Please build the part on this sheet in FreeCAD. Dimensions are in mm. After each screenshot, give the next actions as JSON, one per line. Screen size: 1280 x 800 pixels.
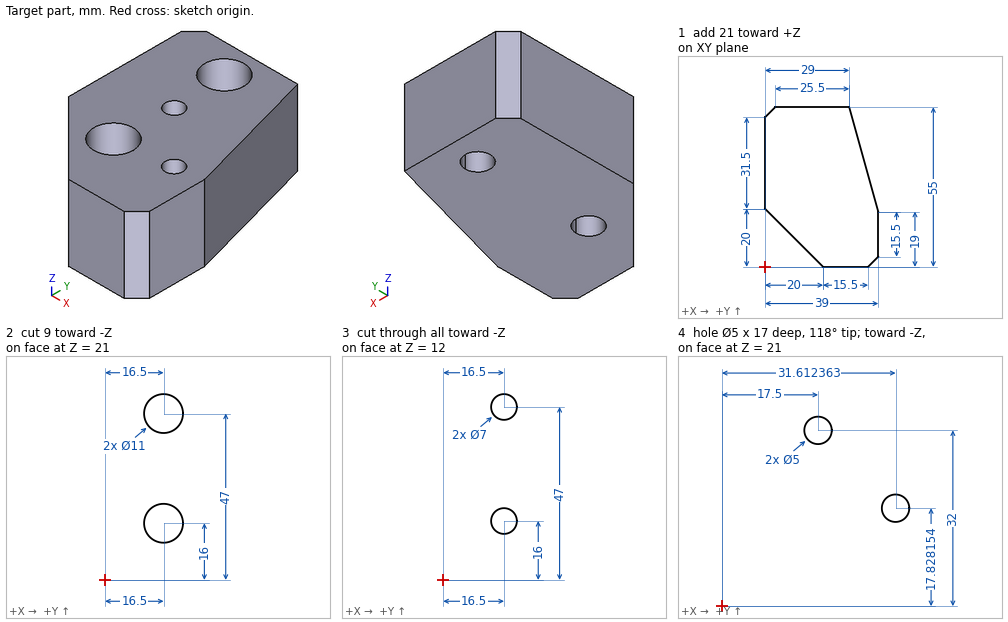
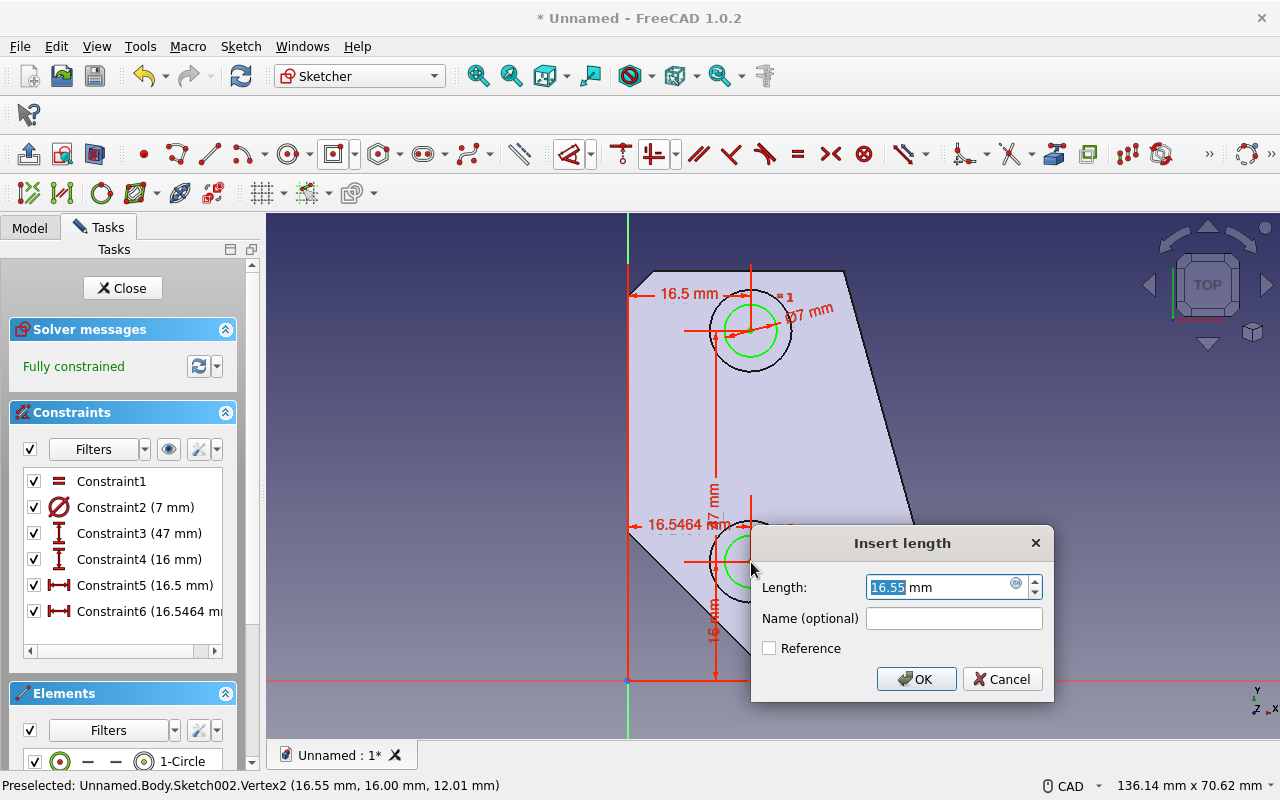
{"action": "type", "text": "16.5"}
{"action": "key", "text": "Return"}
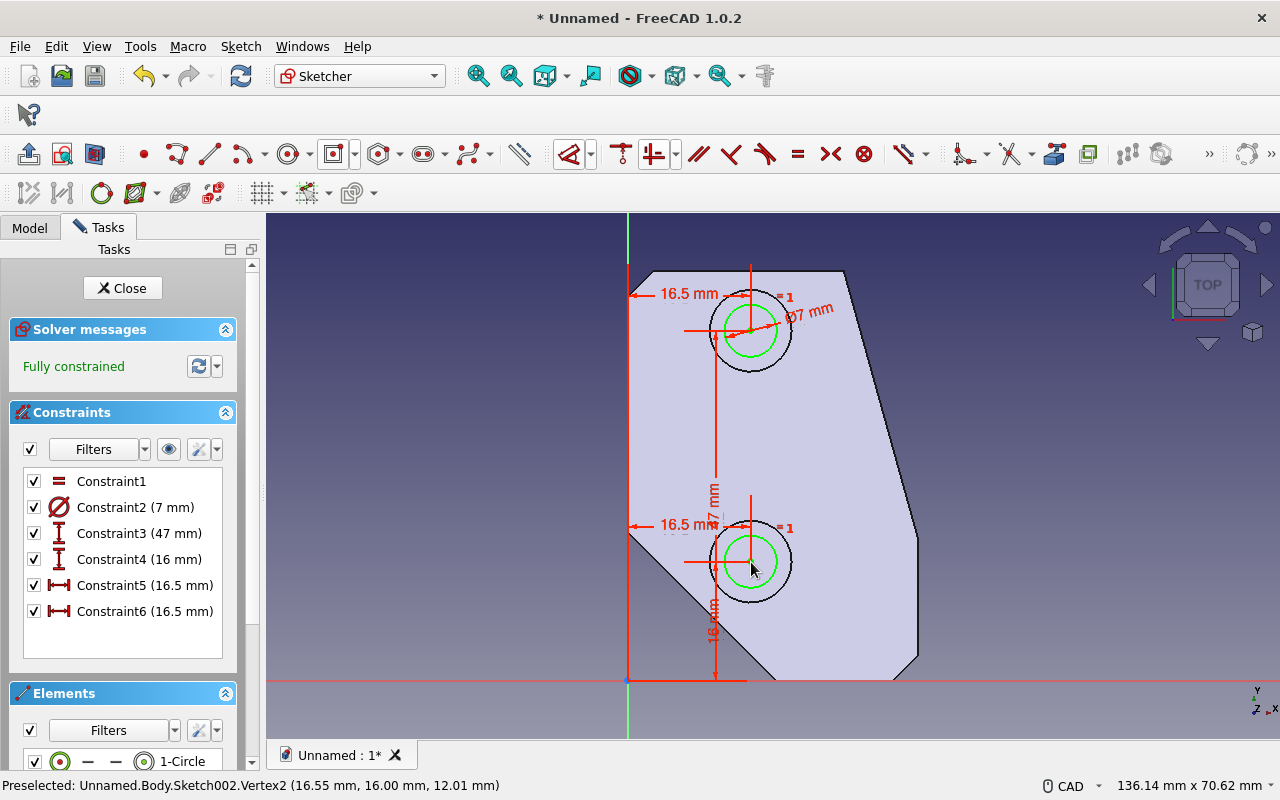
{"action": "left_click", "coordinate": [123, 288]}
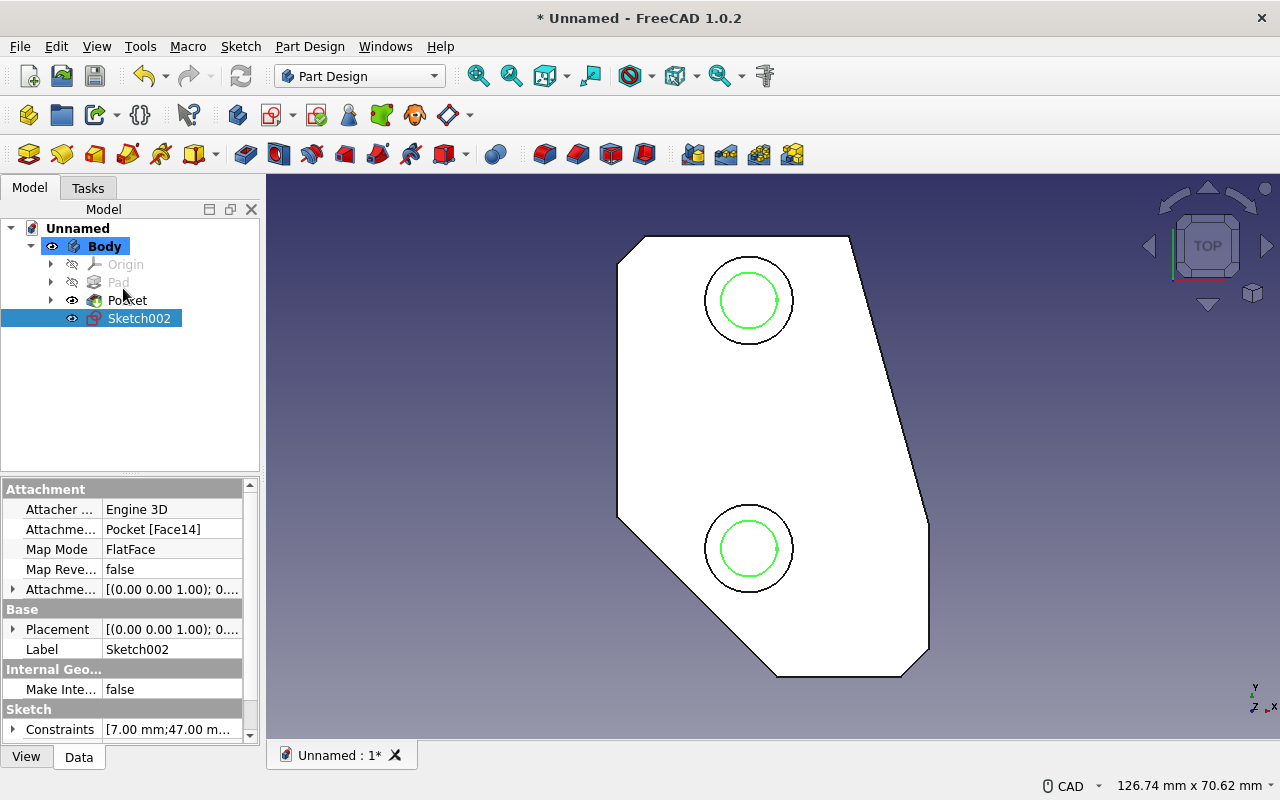
{"action": "left_click", "coordinate": [246, 154]}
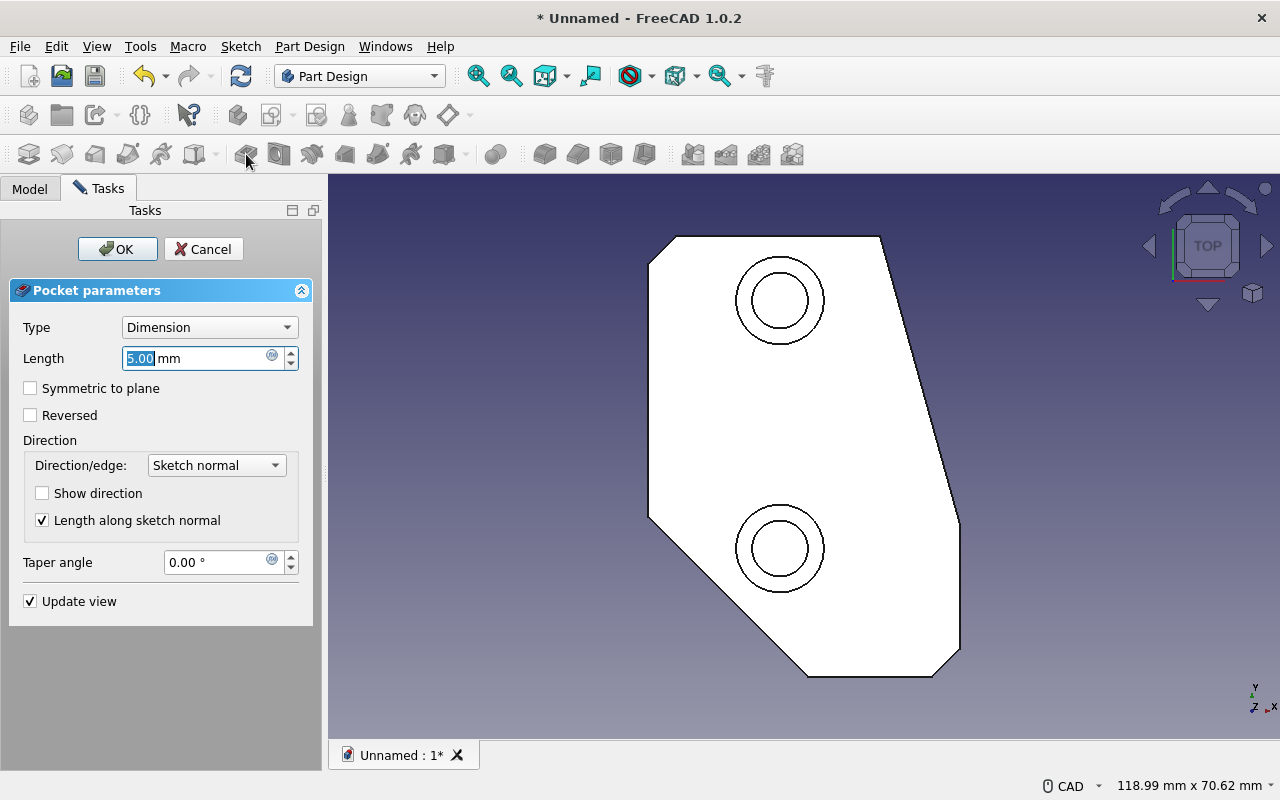
{"action": "left_click", "coordinate": [210, 328]}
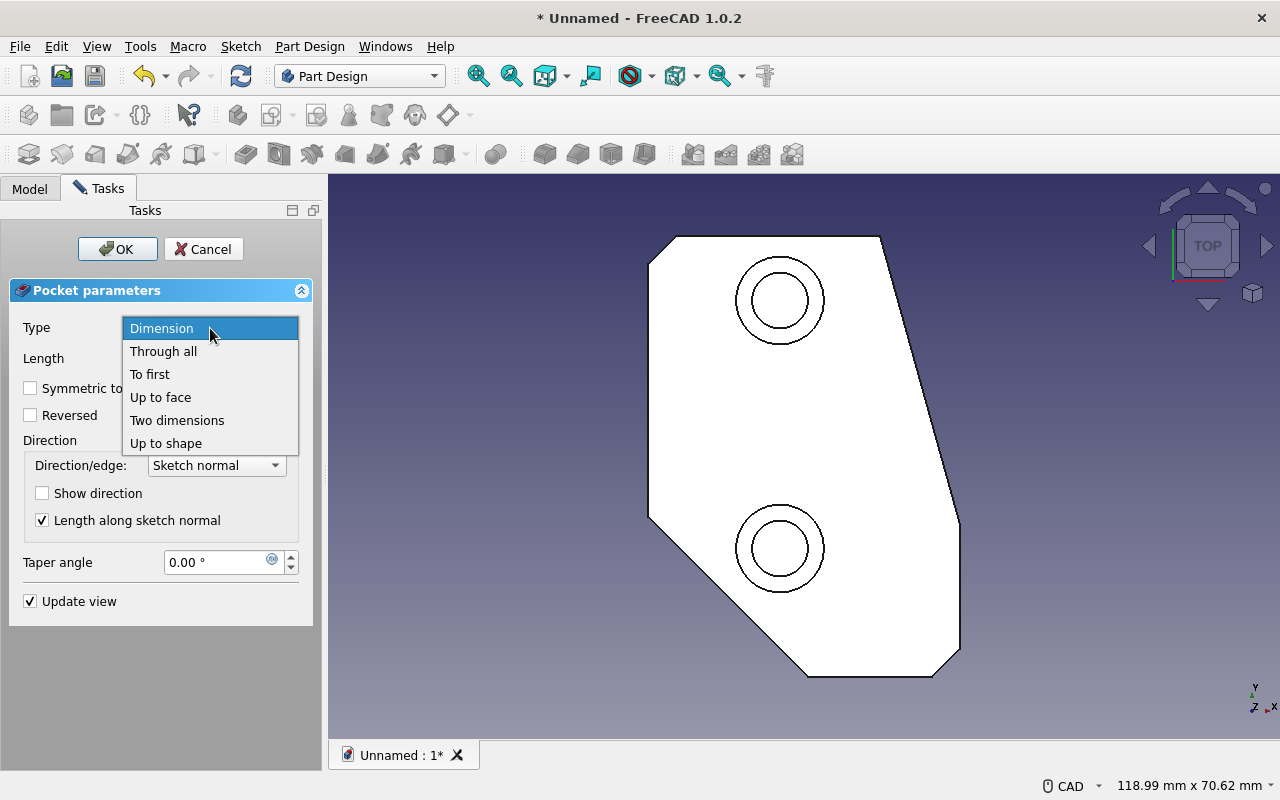
{"action": "left_click", "coordinate": [208, 352]}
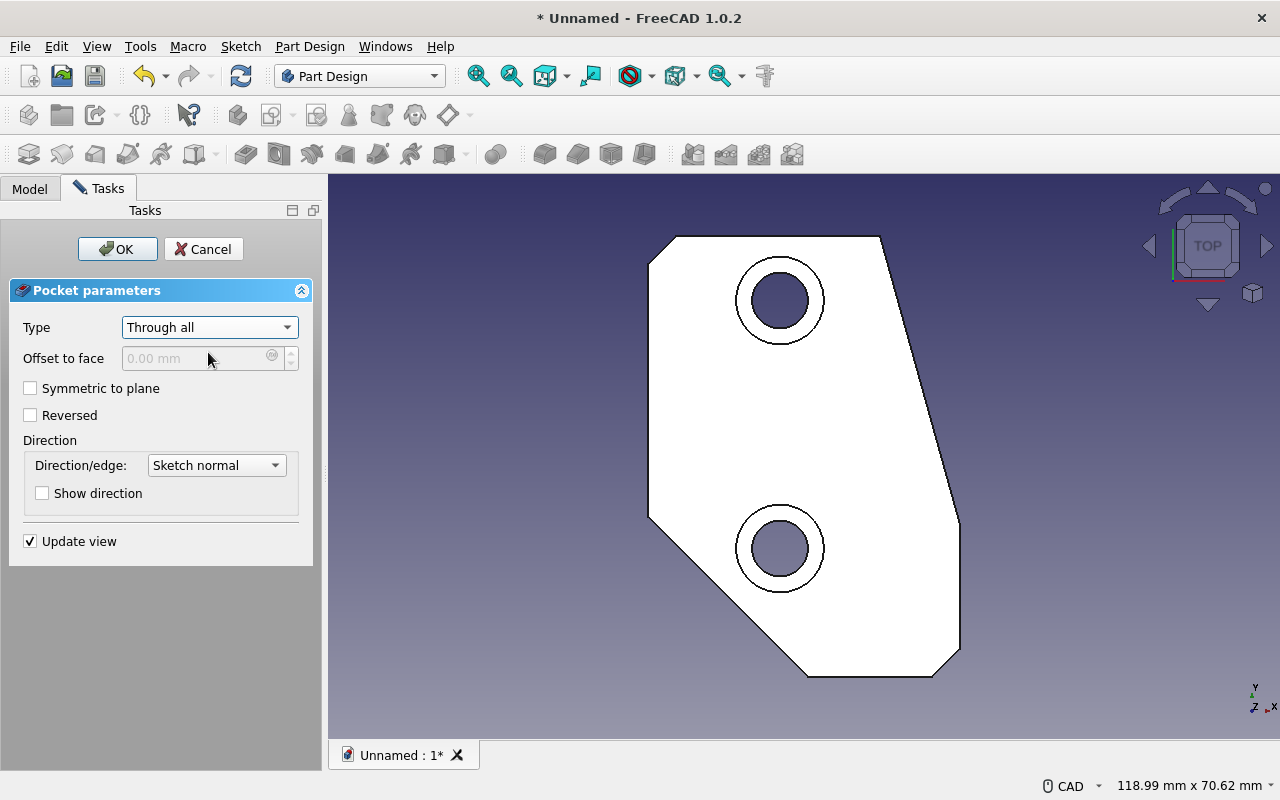
{"action": "left_click", "coordinate": [118, 249]}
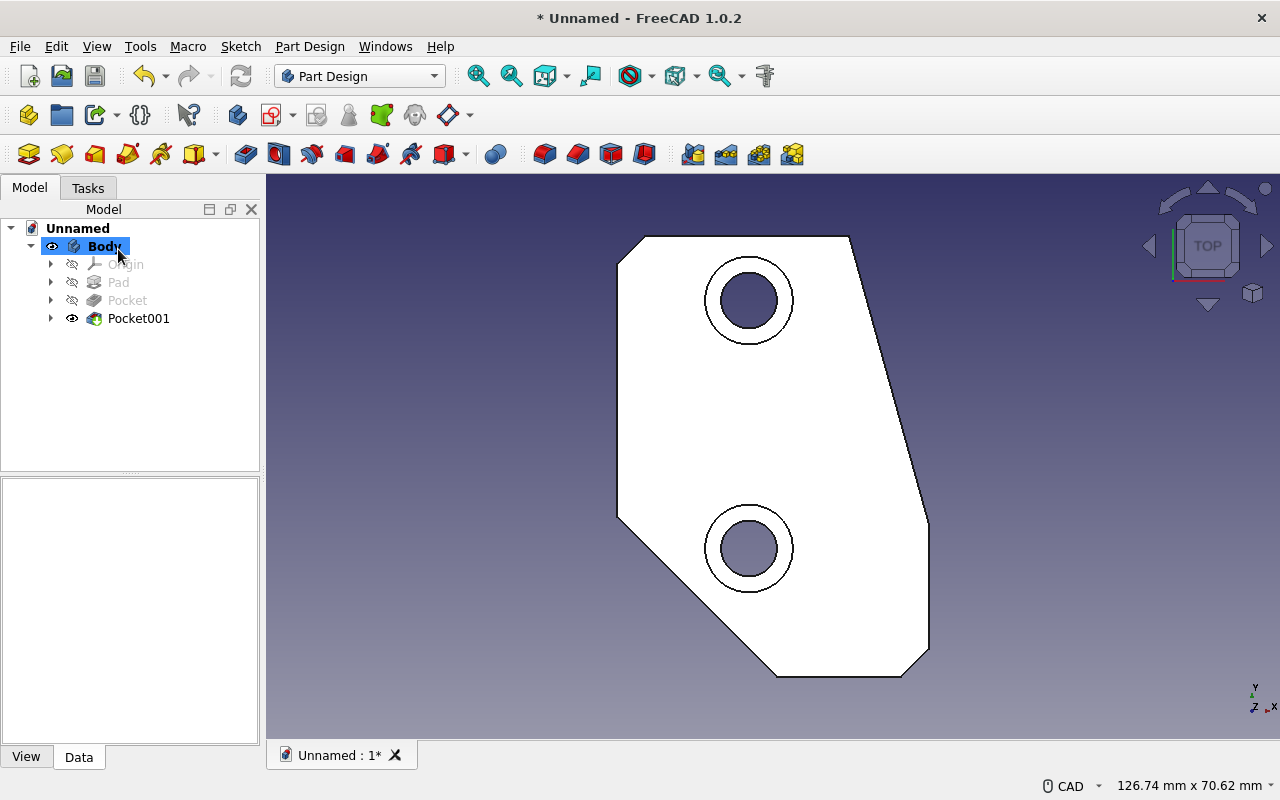
{"action": "left_click", "coordinate": [818, 393]}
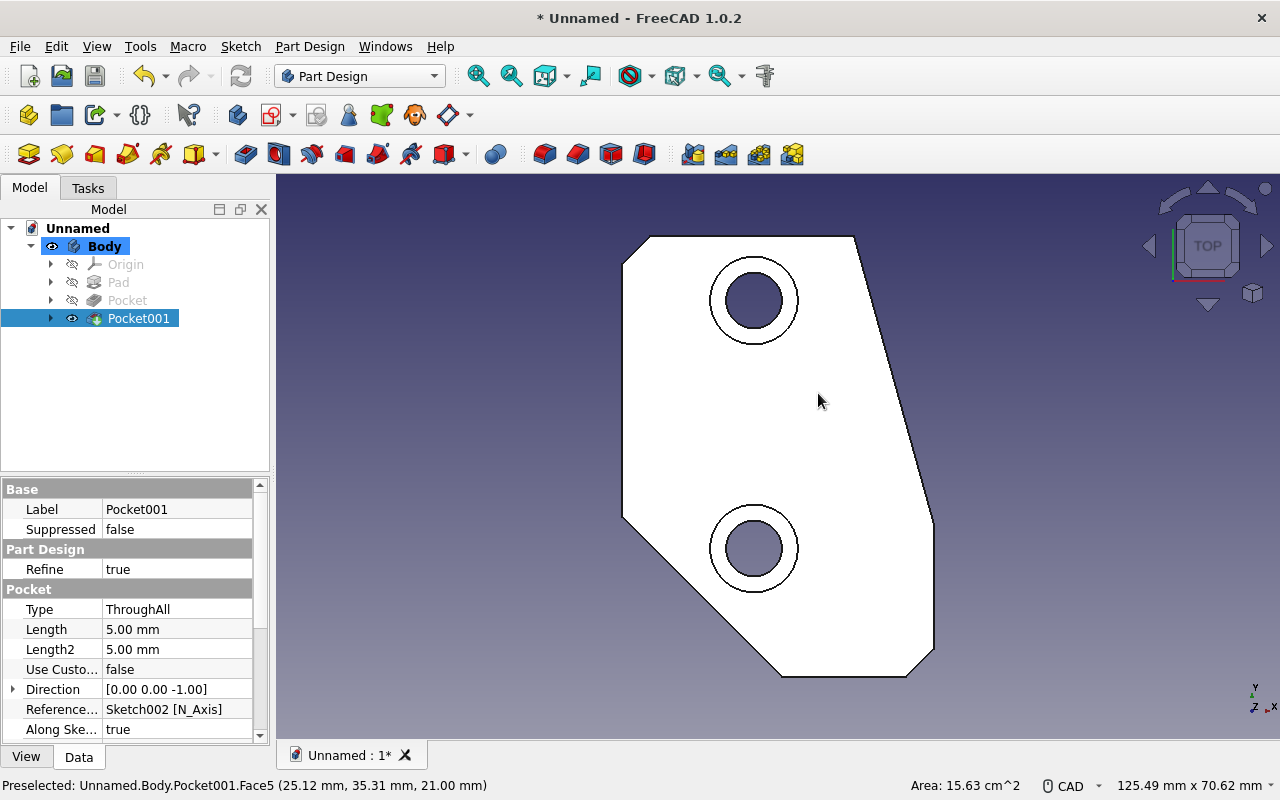
{"action": "left_click", "coordinate": [270, 116]}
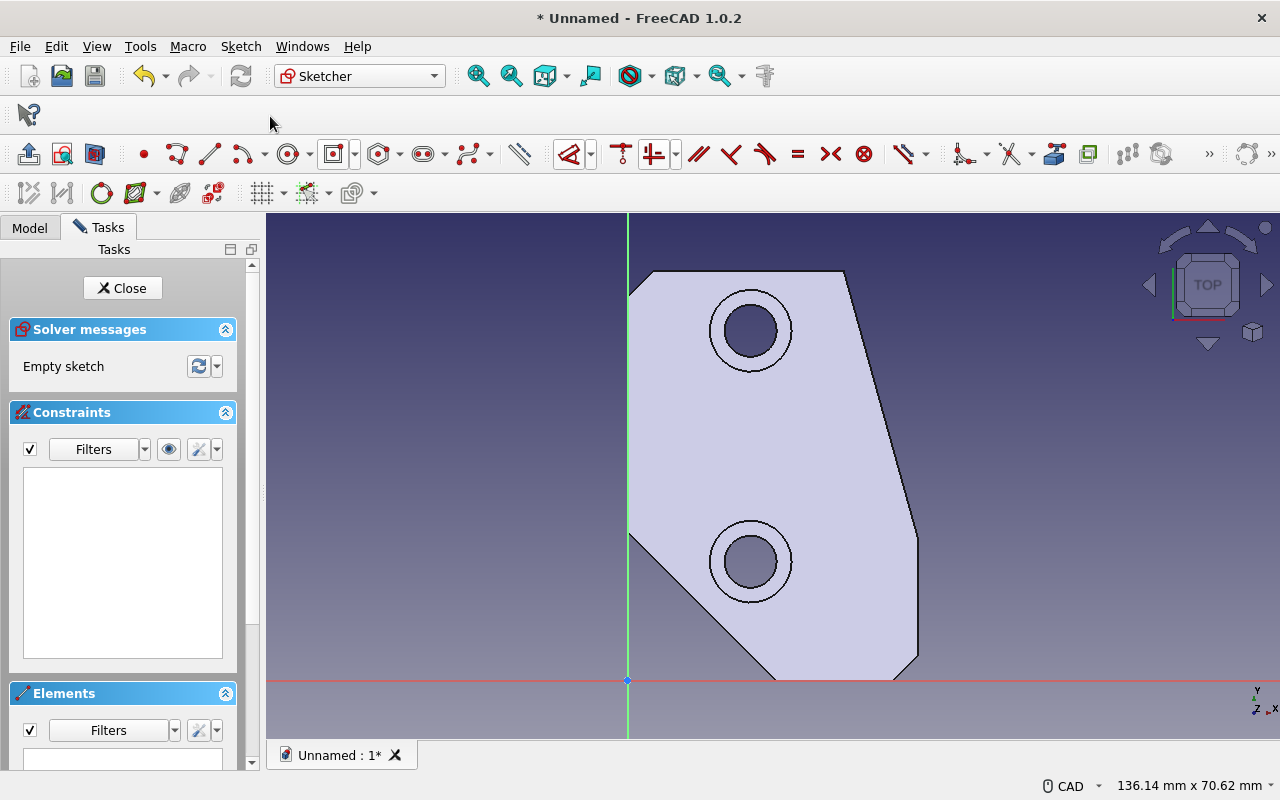
{"action": "left_click", "coordinate": [288, 154]}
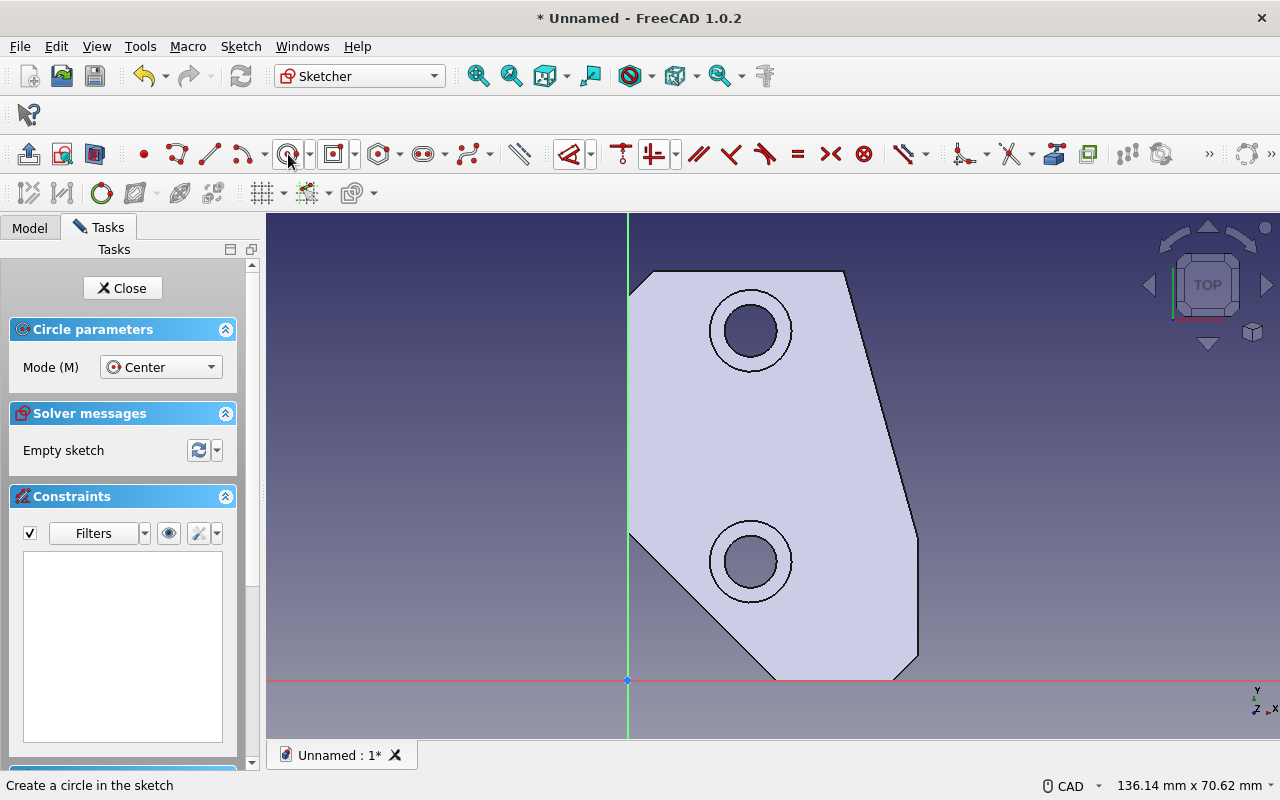
{"action": "left_click", "coordinate": [758, 442]}
{"action": "left_click", "coordinate": [771, 429]}